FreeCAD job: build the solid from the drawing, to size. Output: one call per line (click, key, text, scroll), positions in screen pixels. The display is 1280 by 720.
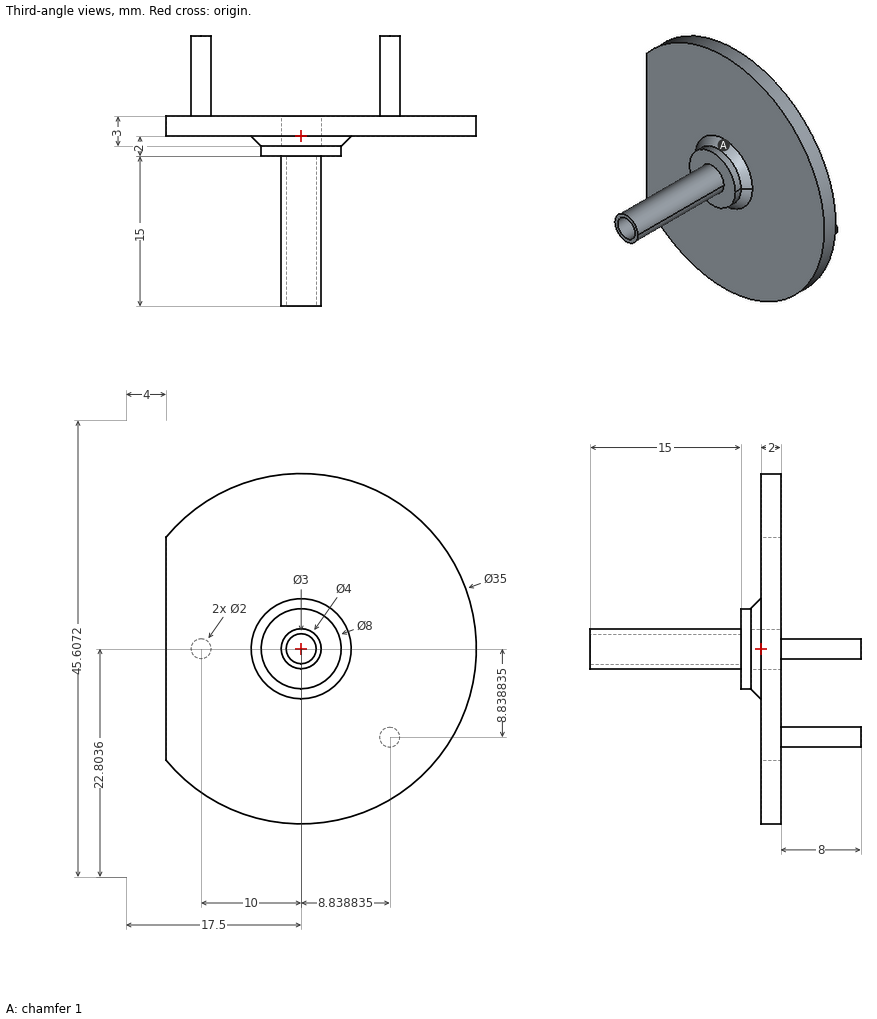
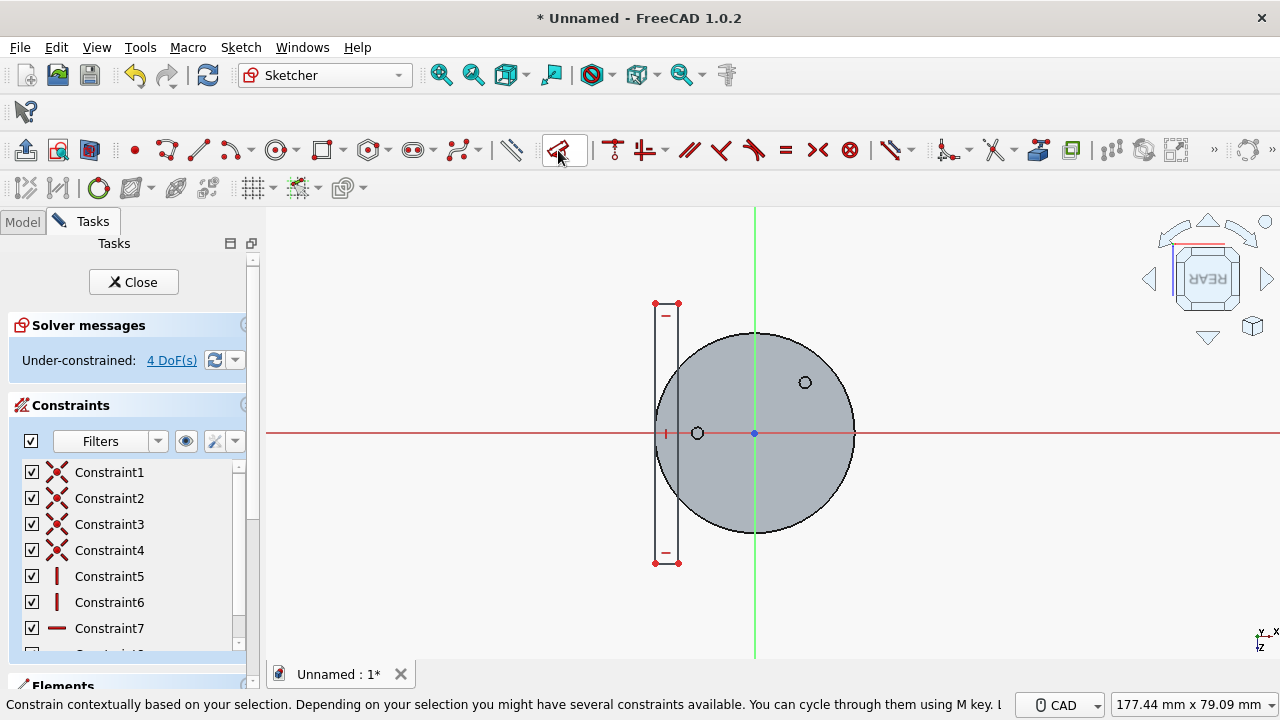
scroll(664, 564, up, 3)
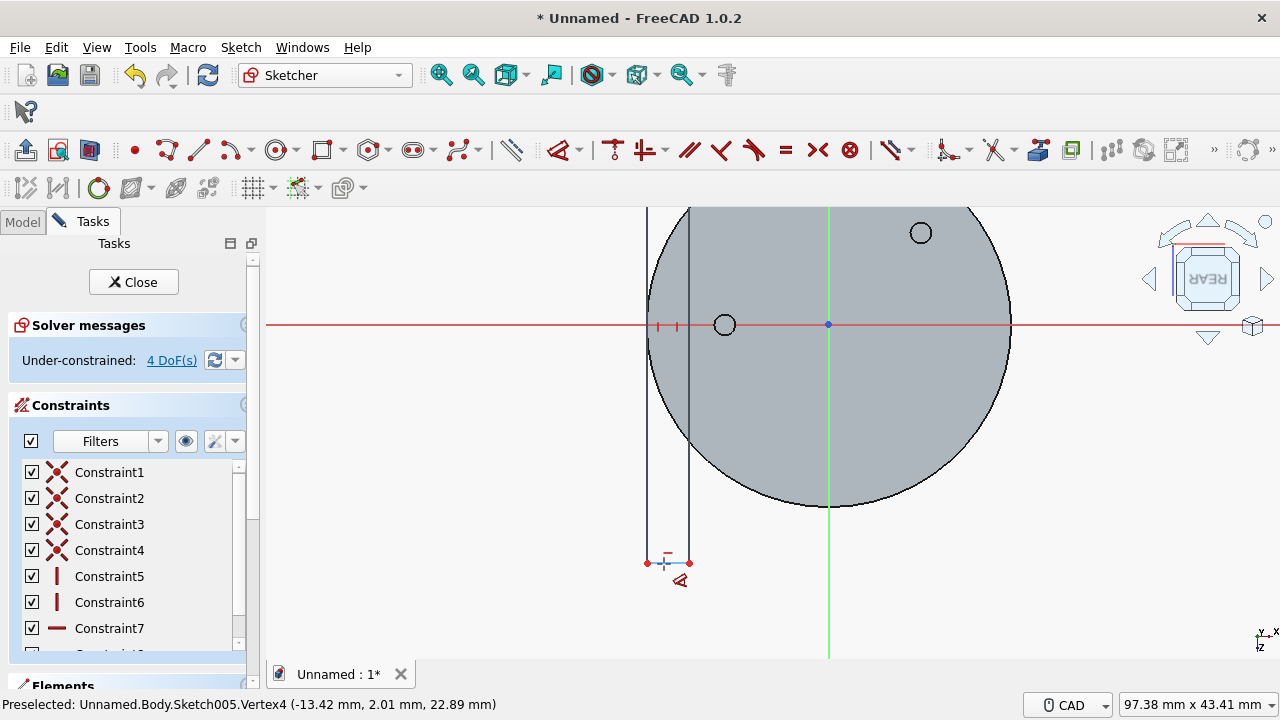
click(664, 563)
click(668, 597)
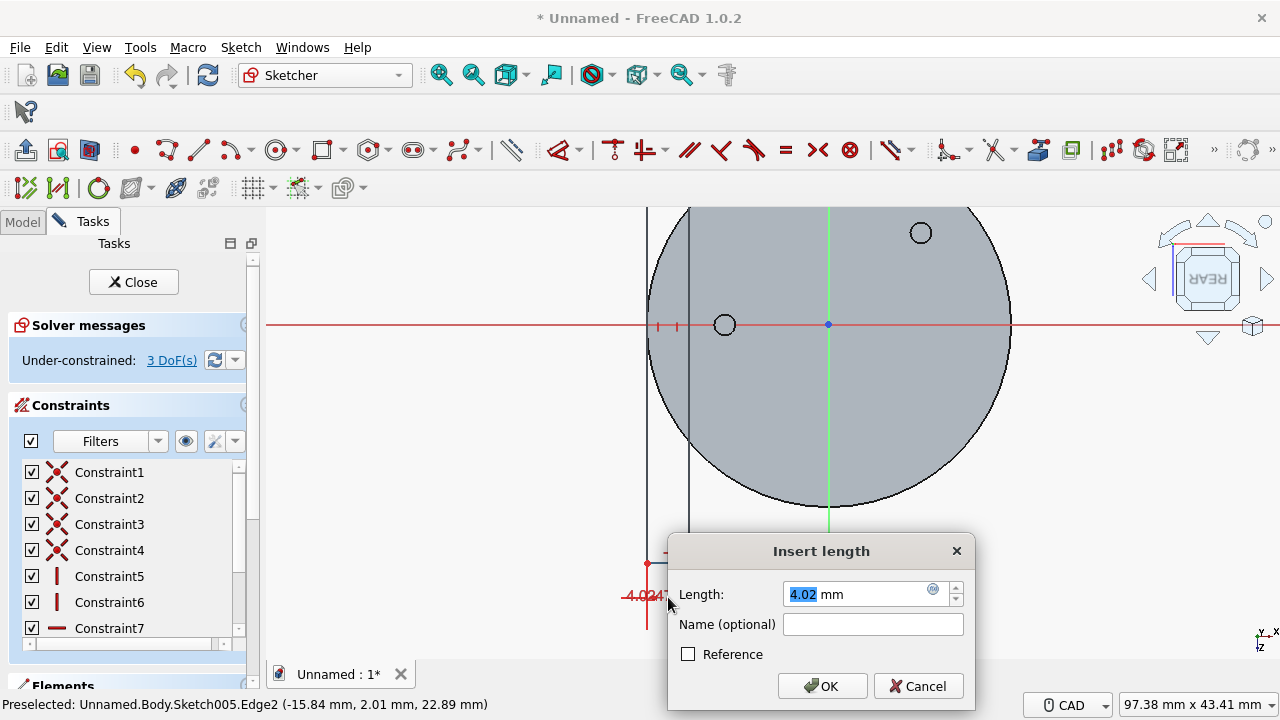
text(4)
key(Return)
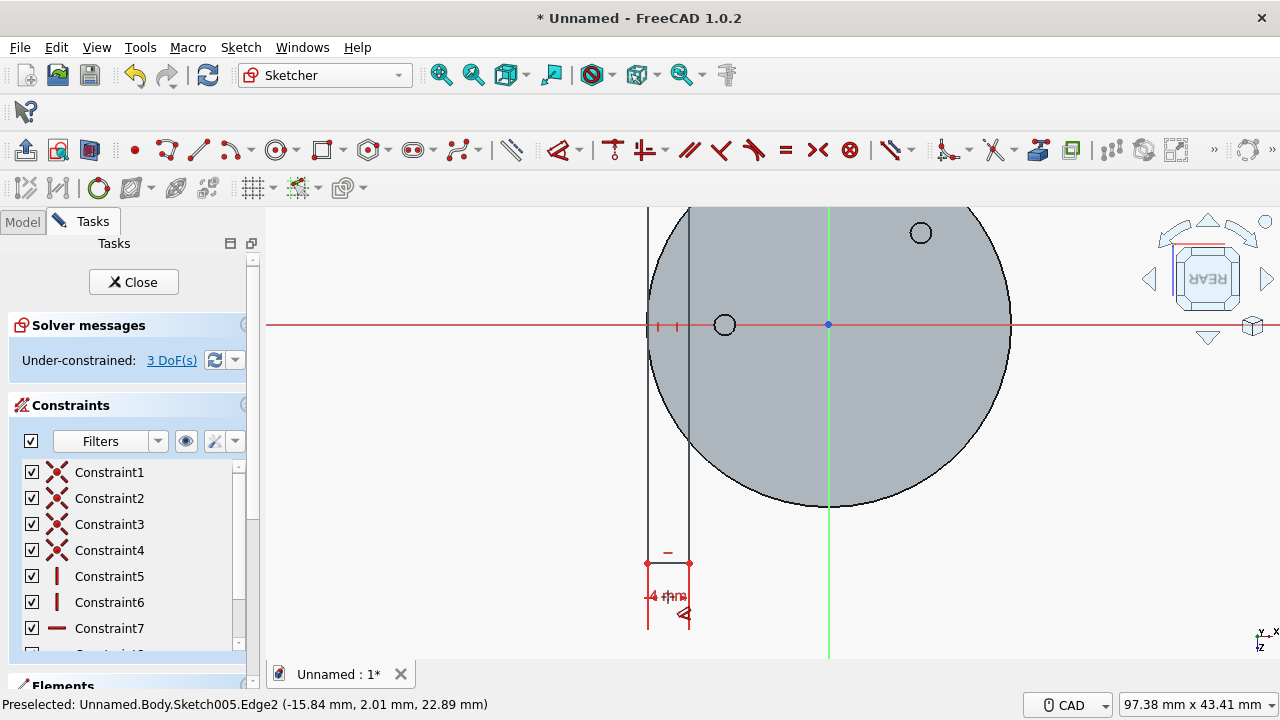
scroll(664, 564, down, 3)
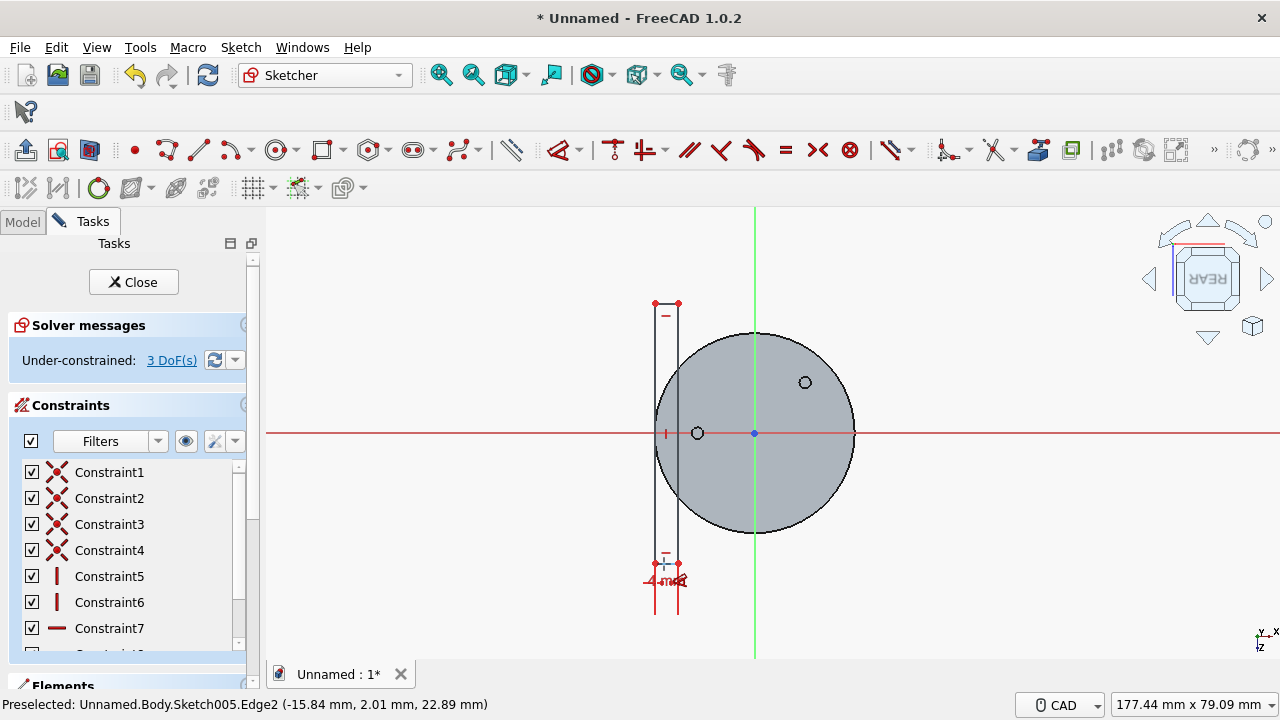
click(655, 304)
click(705, 270)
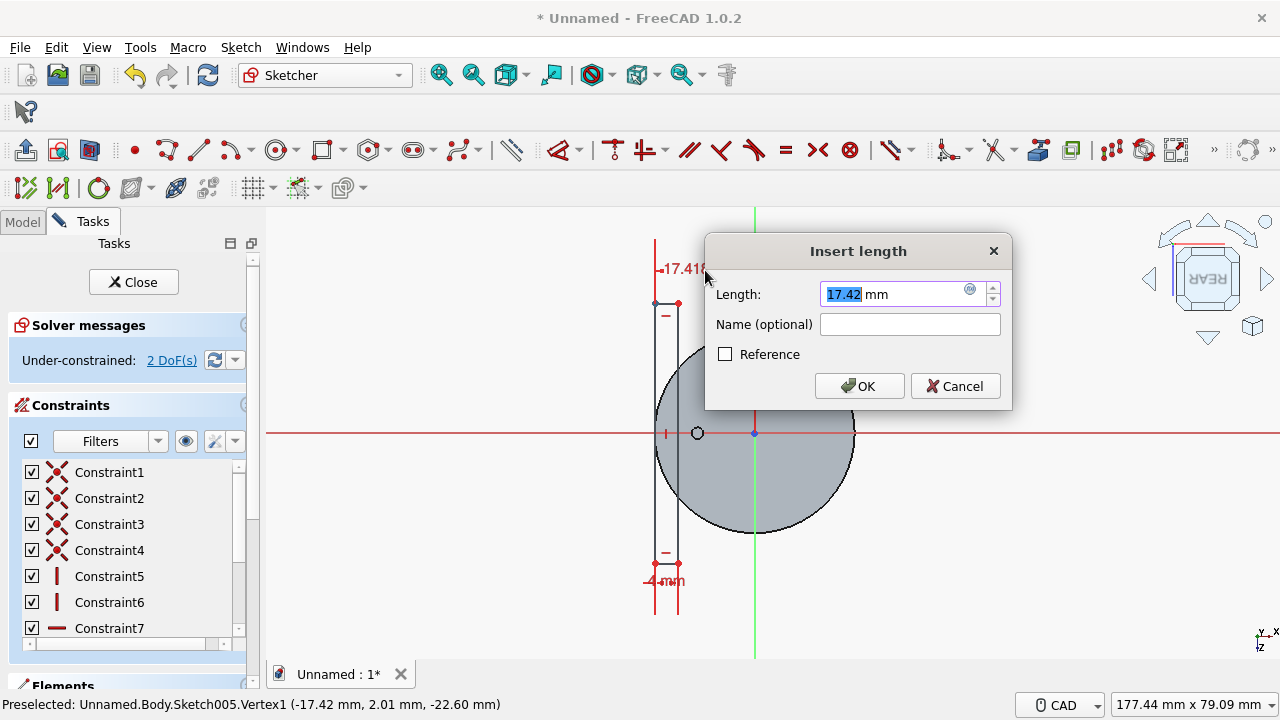
text(17.5)
key(Return)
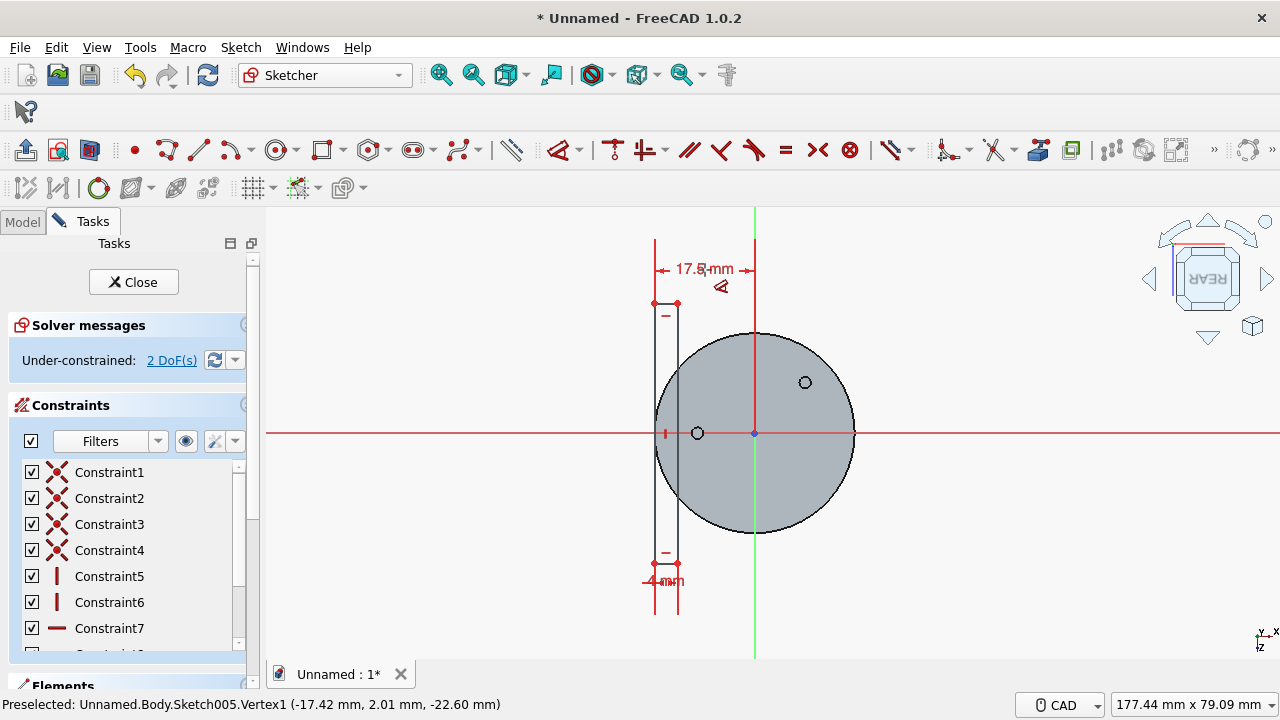
click(655, 382)
click(621, 374)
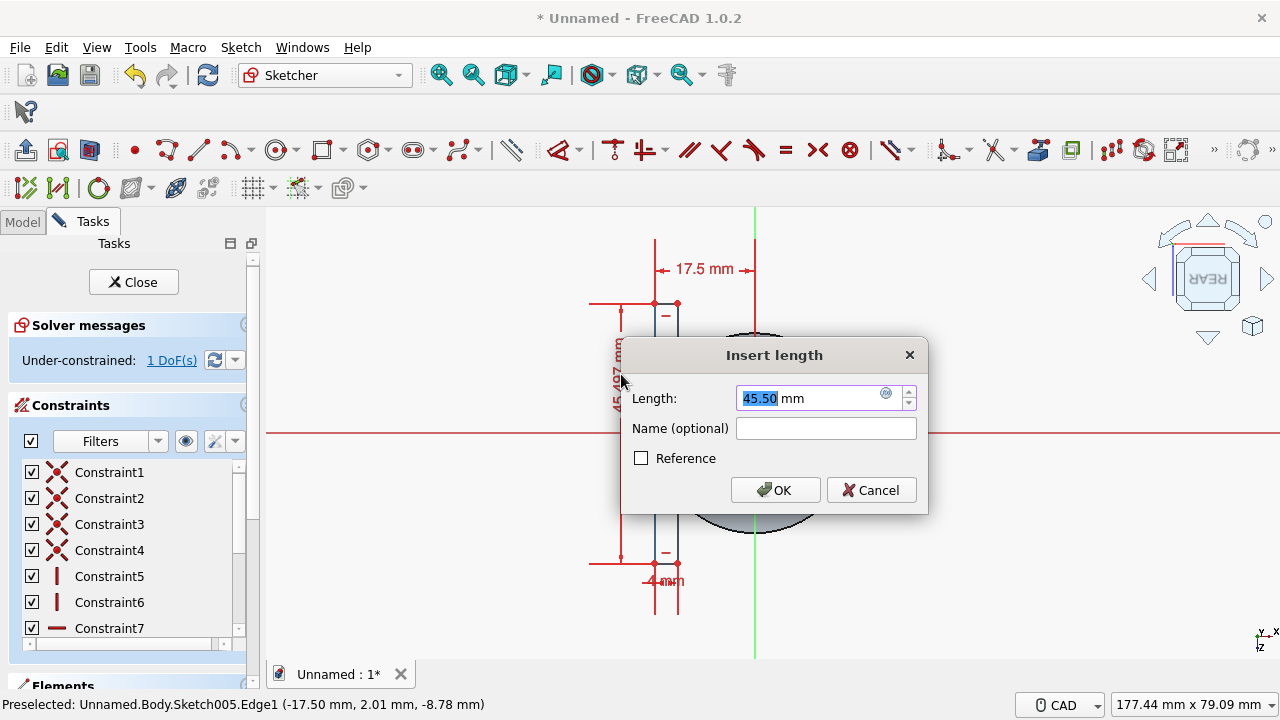
text(45.6072)
key(Return)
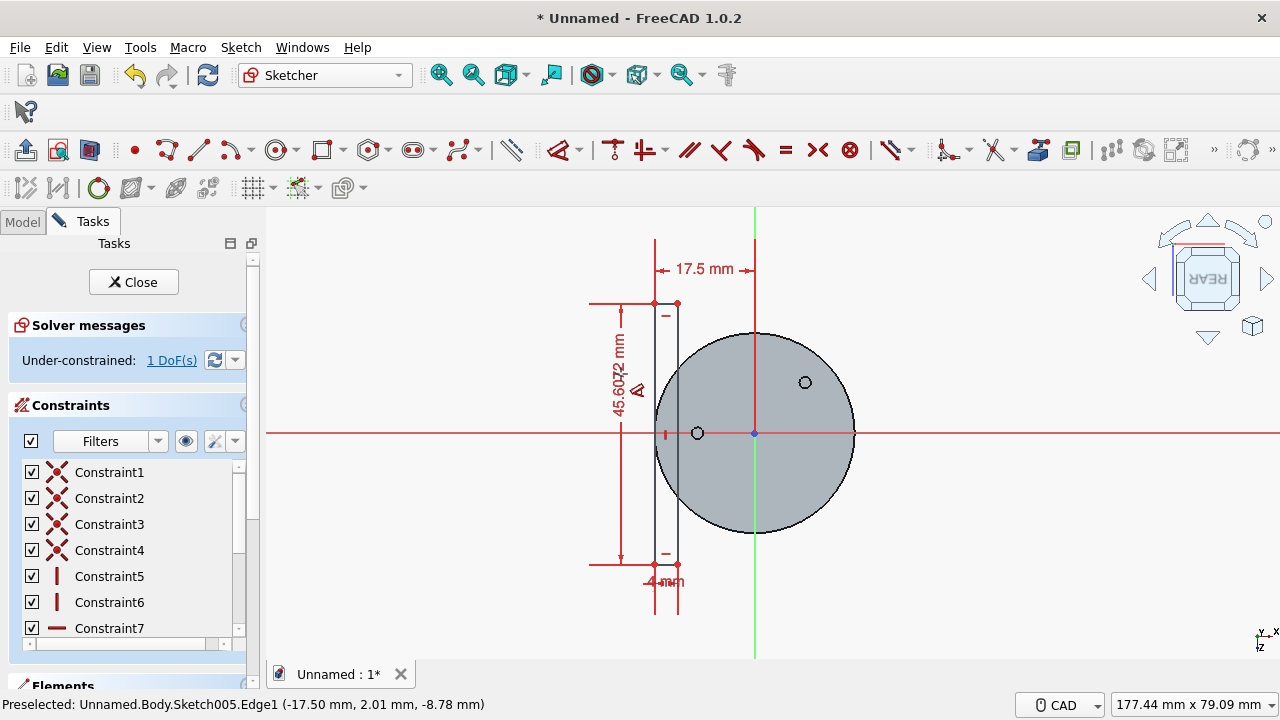
click(655, 304)
click(789, 369)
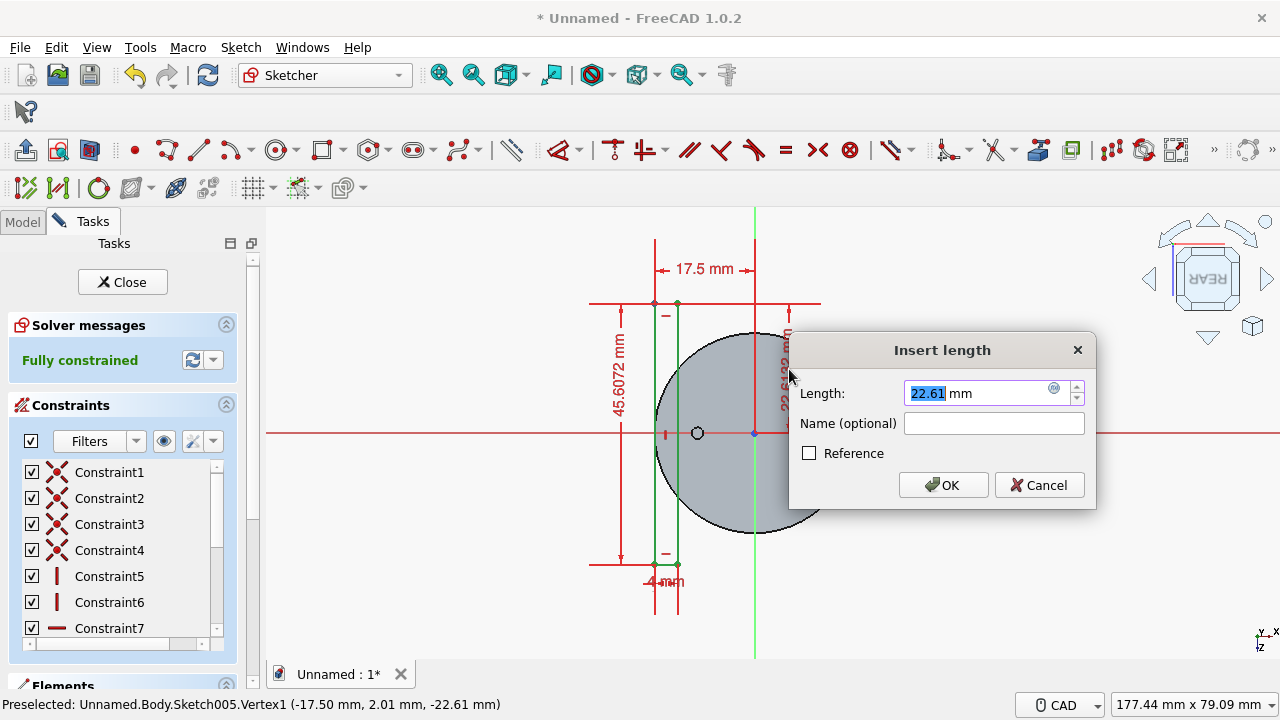
text(22.8036)
key(Return)
key(Escape)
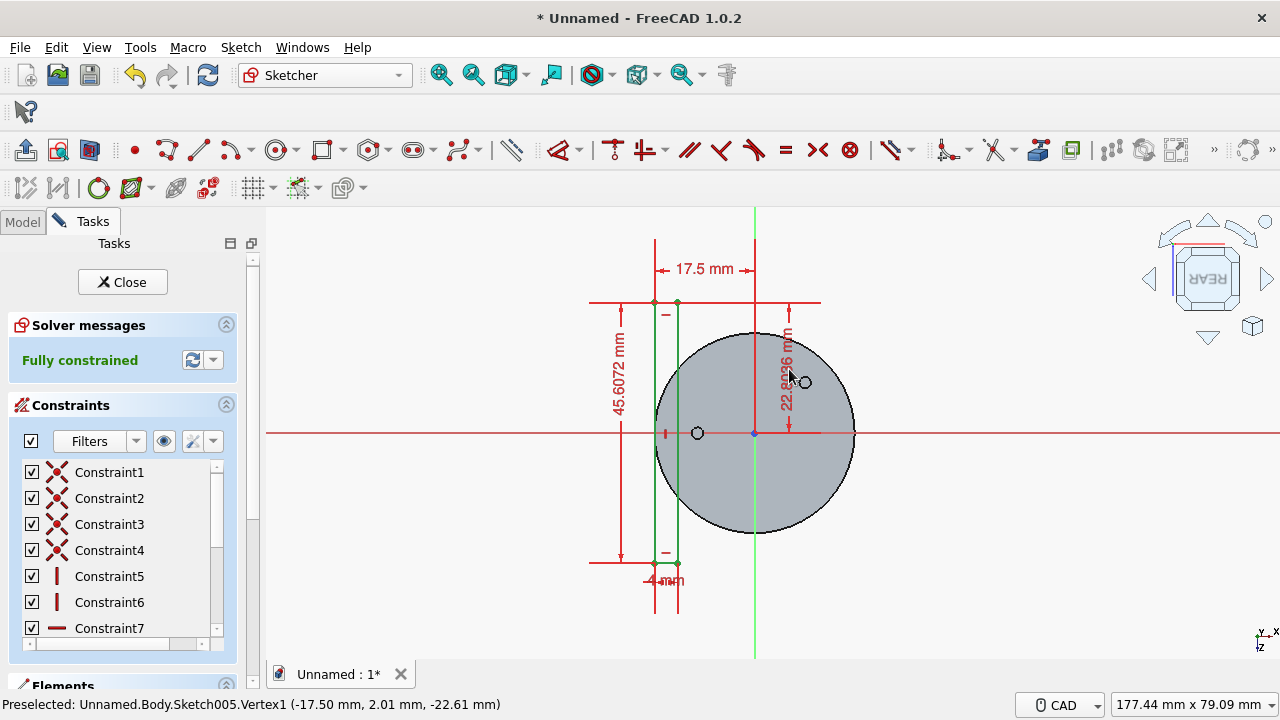
click(123, 282)